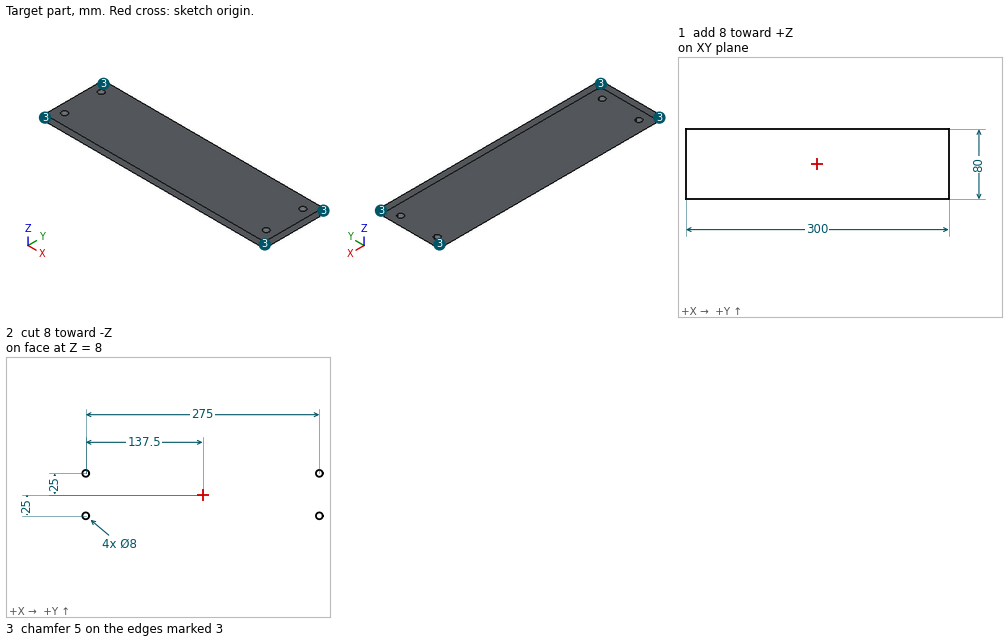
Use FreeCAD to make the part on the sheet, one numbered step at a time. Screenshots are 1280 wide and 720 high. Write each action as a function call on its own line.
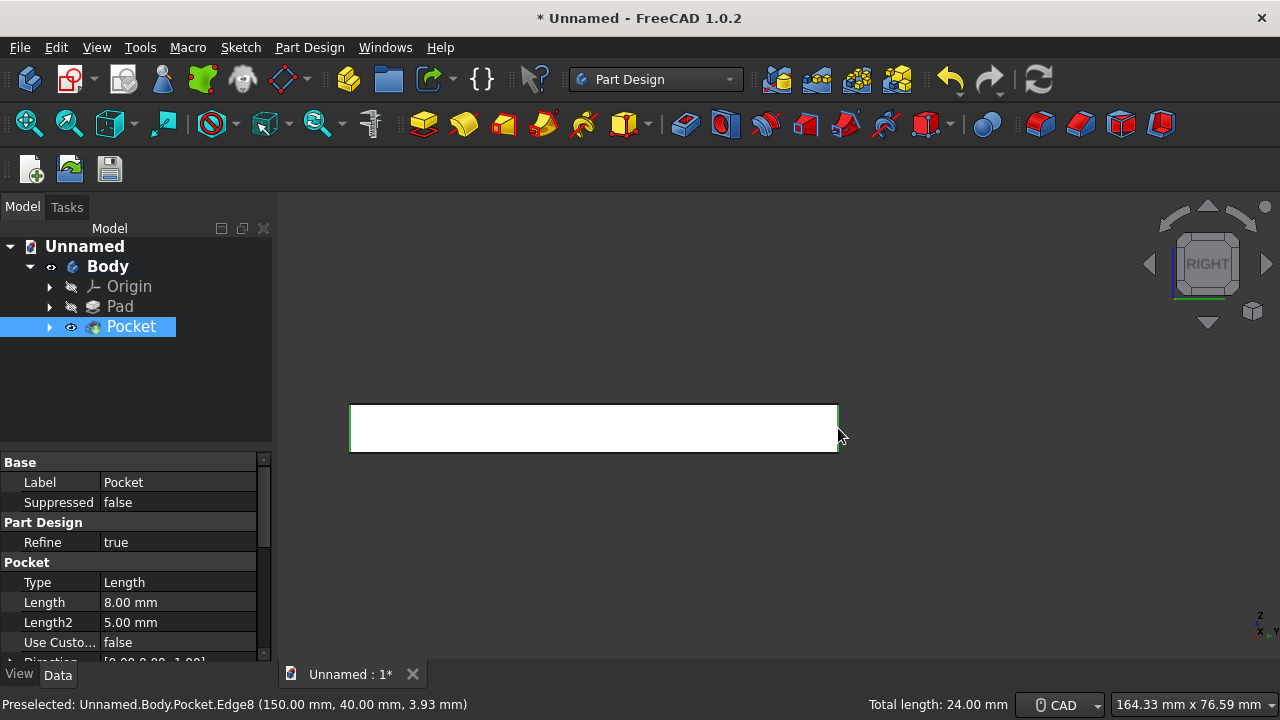
key(v)
key(f)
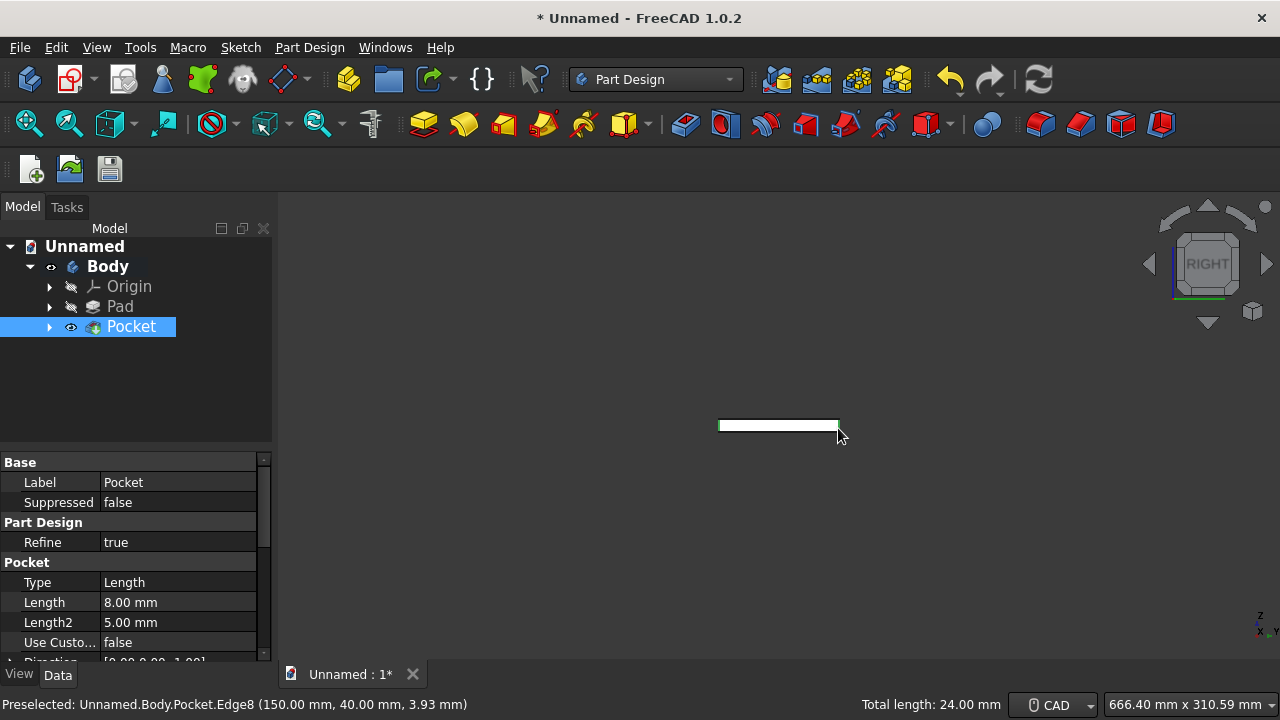
key(5)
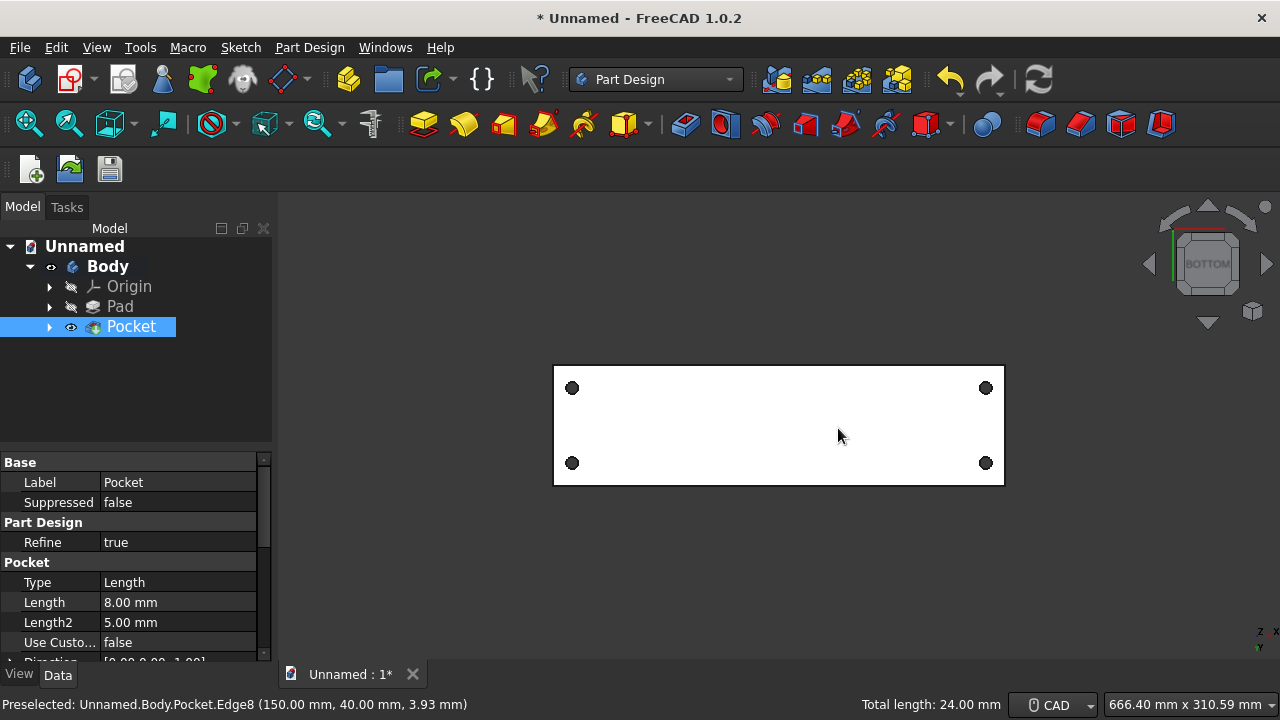
scroll(553, 485, up, 7)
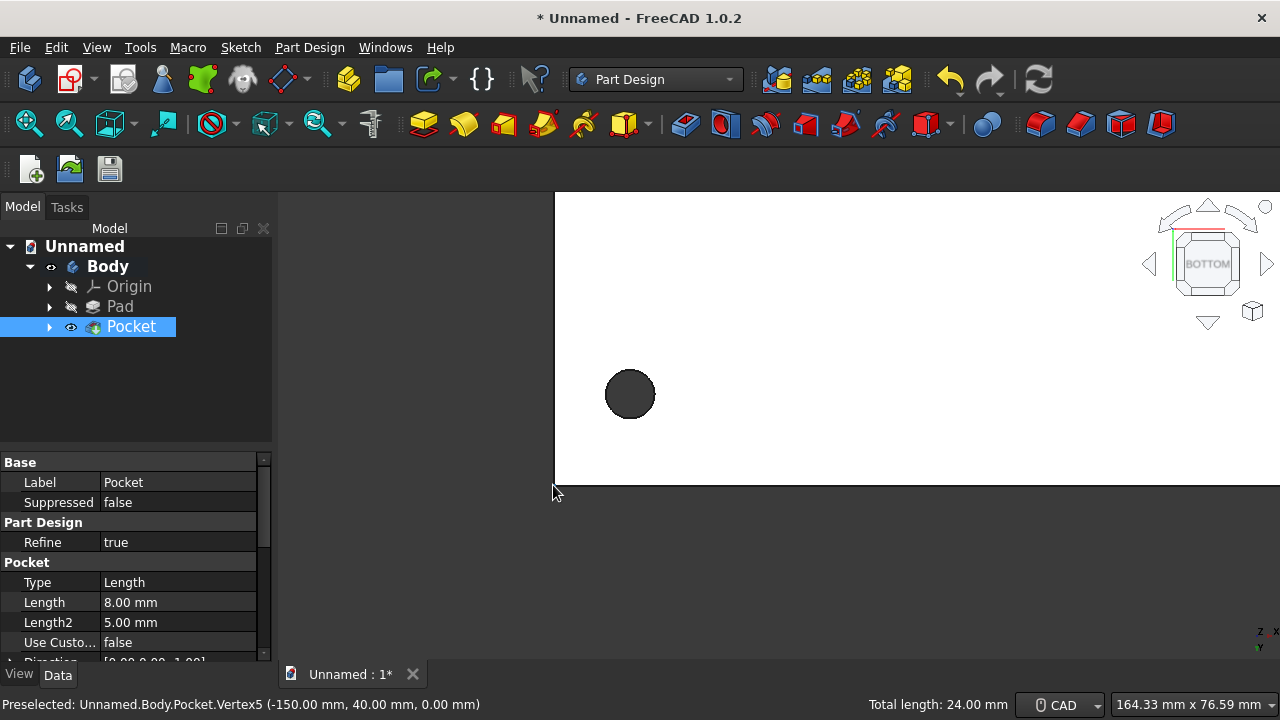
key(v)
key(f)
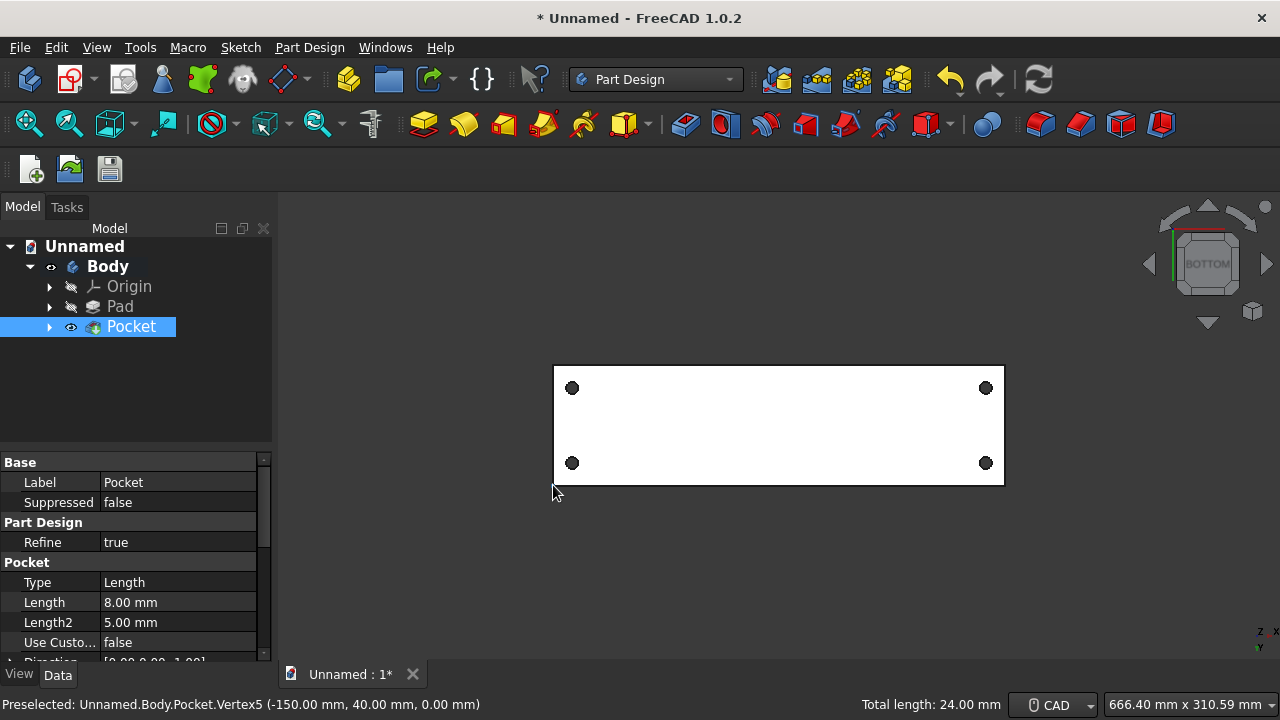
key(4)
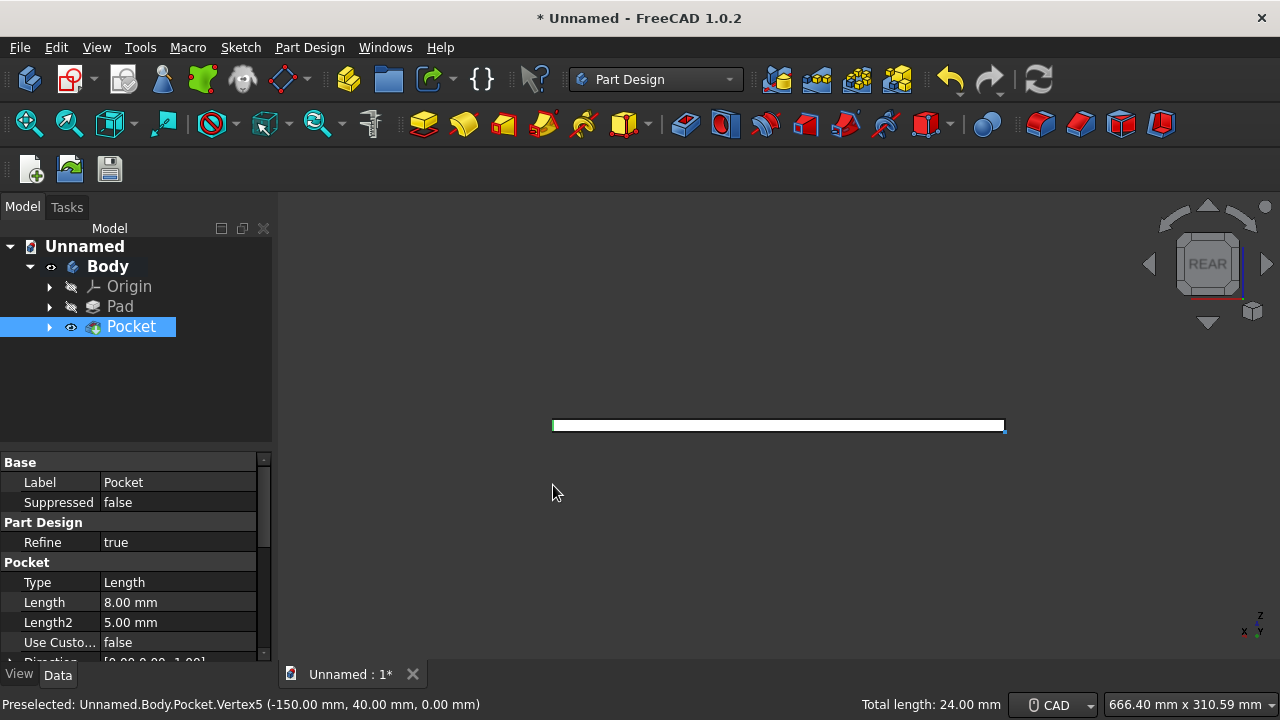
scroll(1005, 425, up, 7)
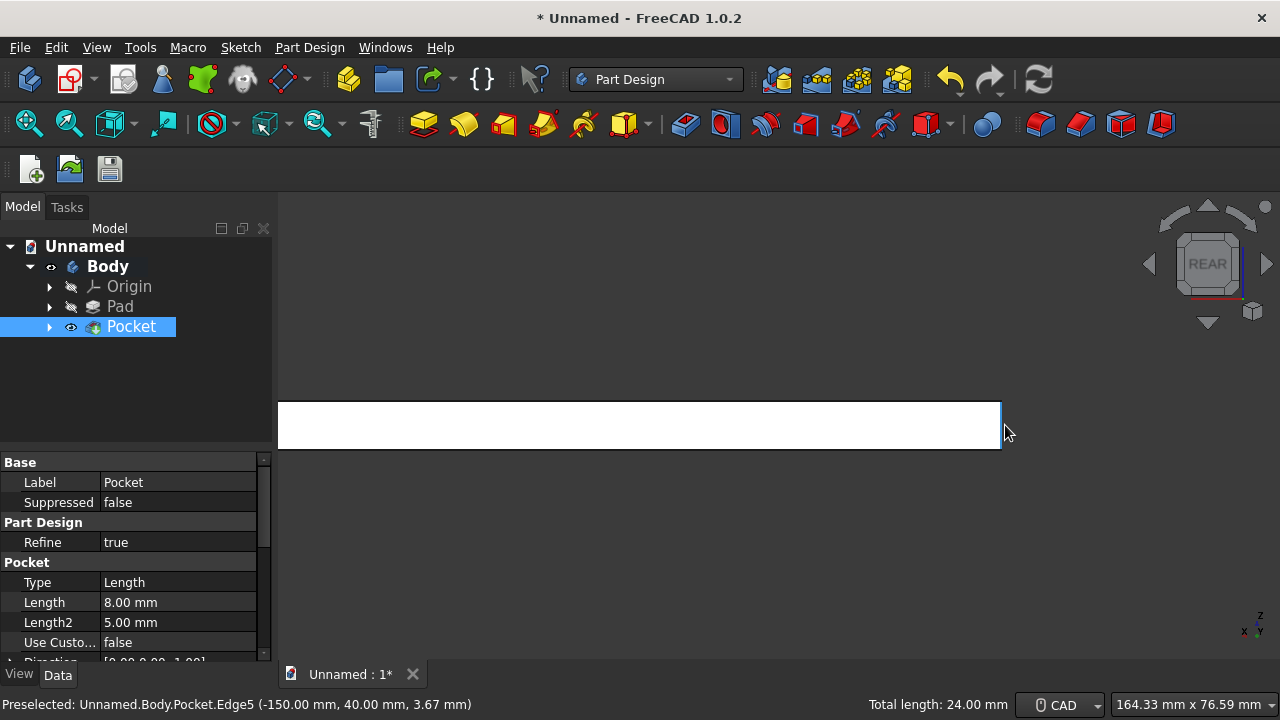
click(1001, 425, ctrl)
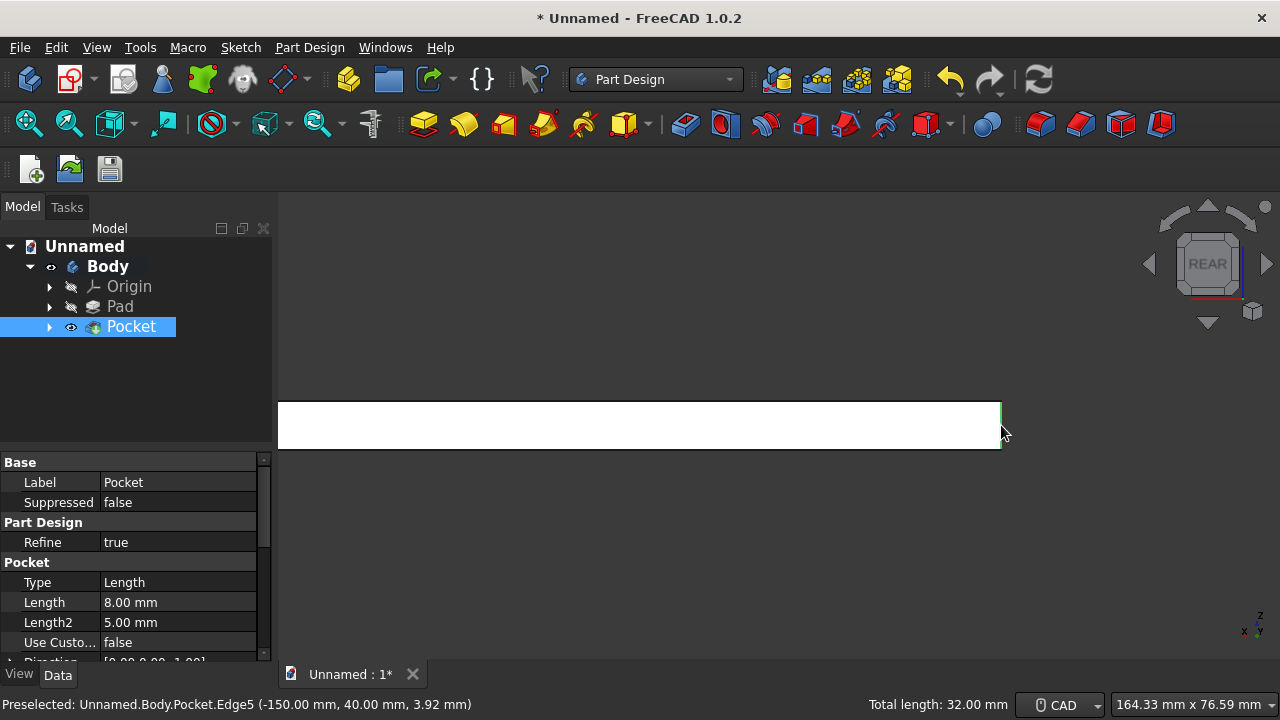
click(1082, 124)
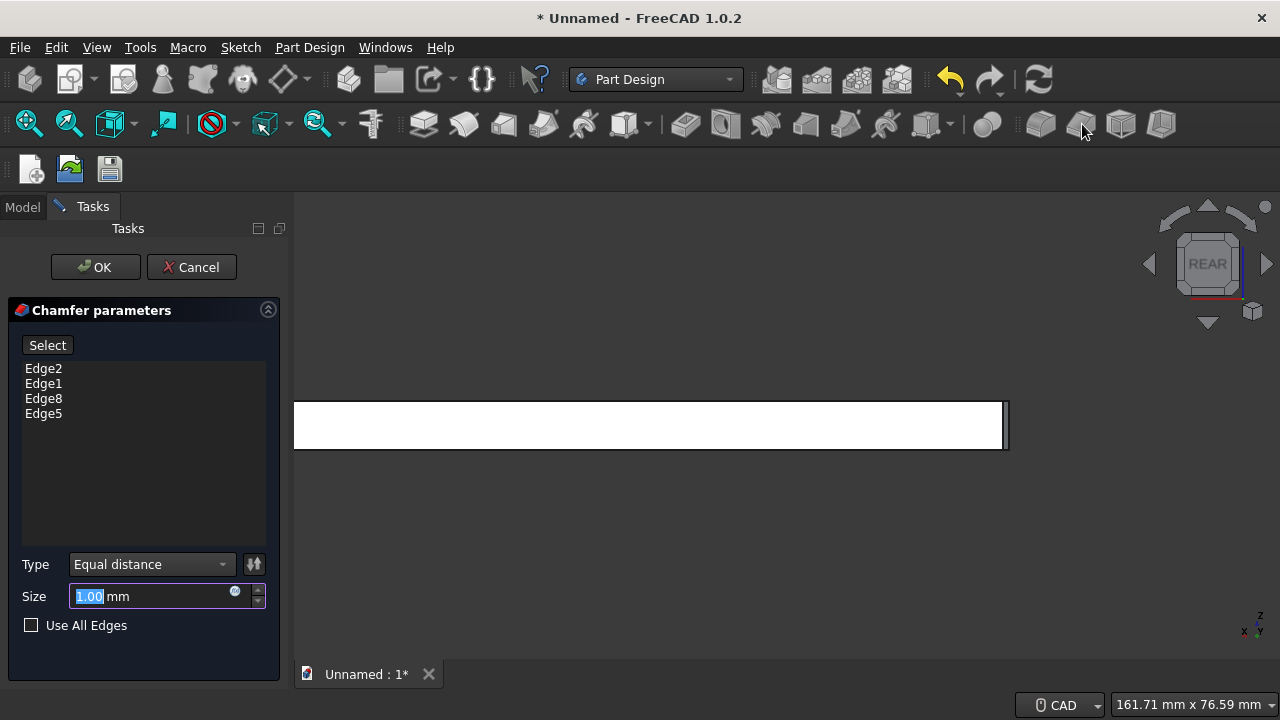
text(5)
key(Tab)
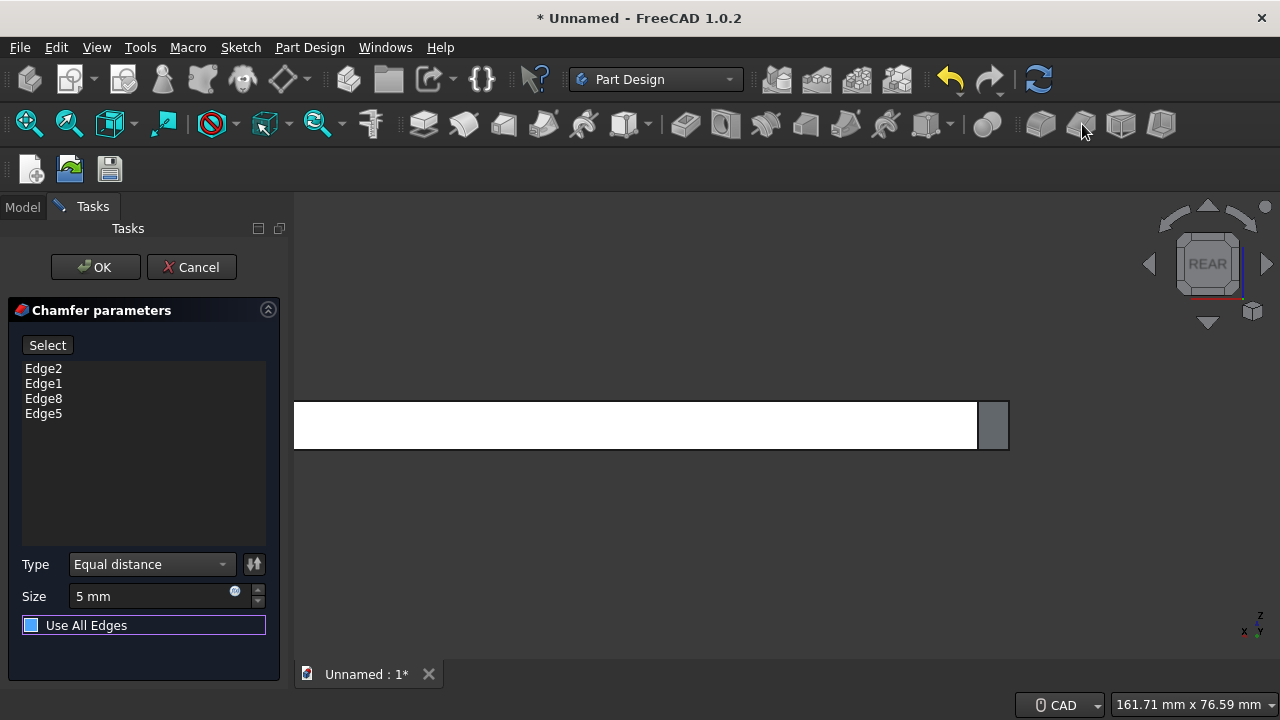
click(96, 267)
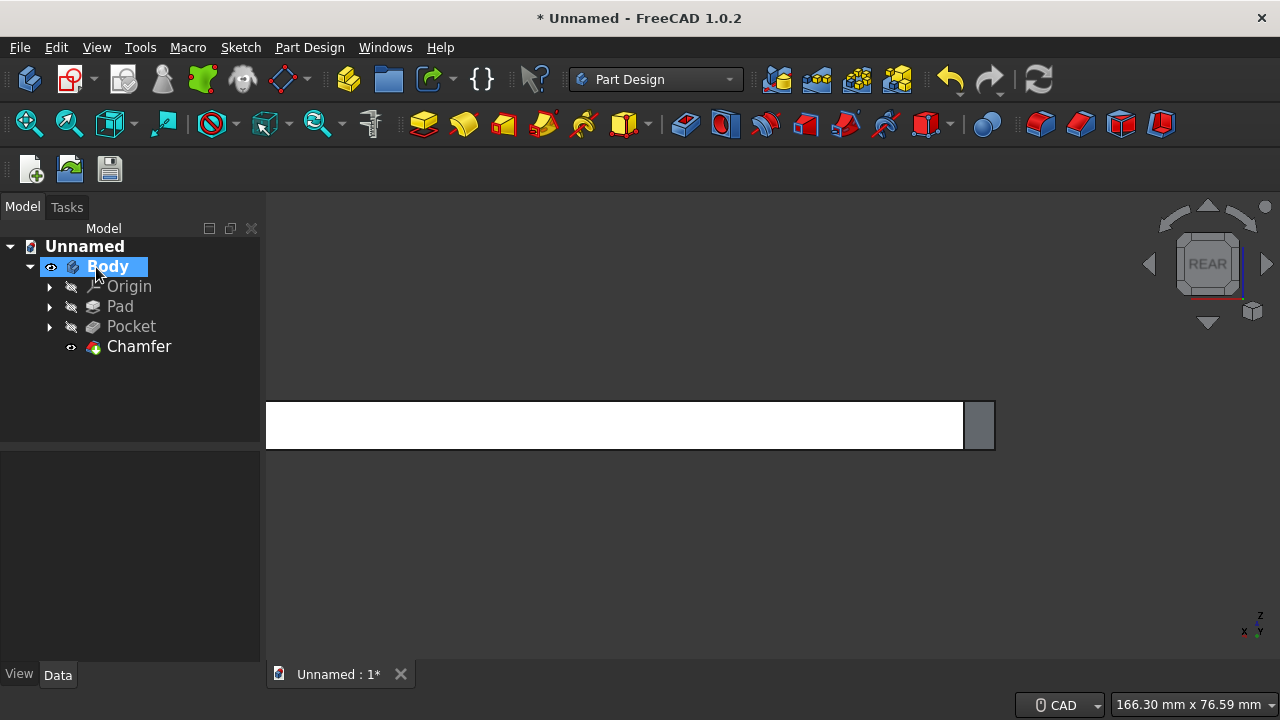
key(0)